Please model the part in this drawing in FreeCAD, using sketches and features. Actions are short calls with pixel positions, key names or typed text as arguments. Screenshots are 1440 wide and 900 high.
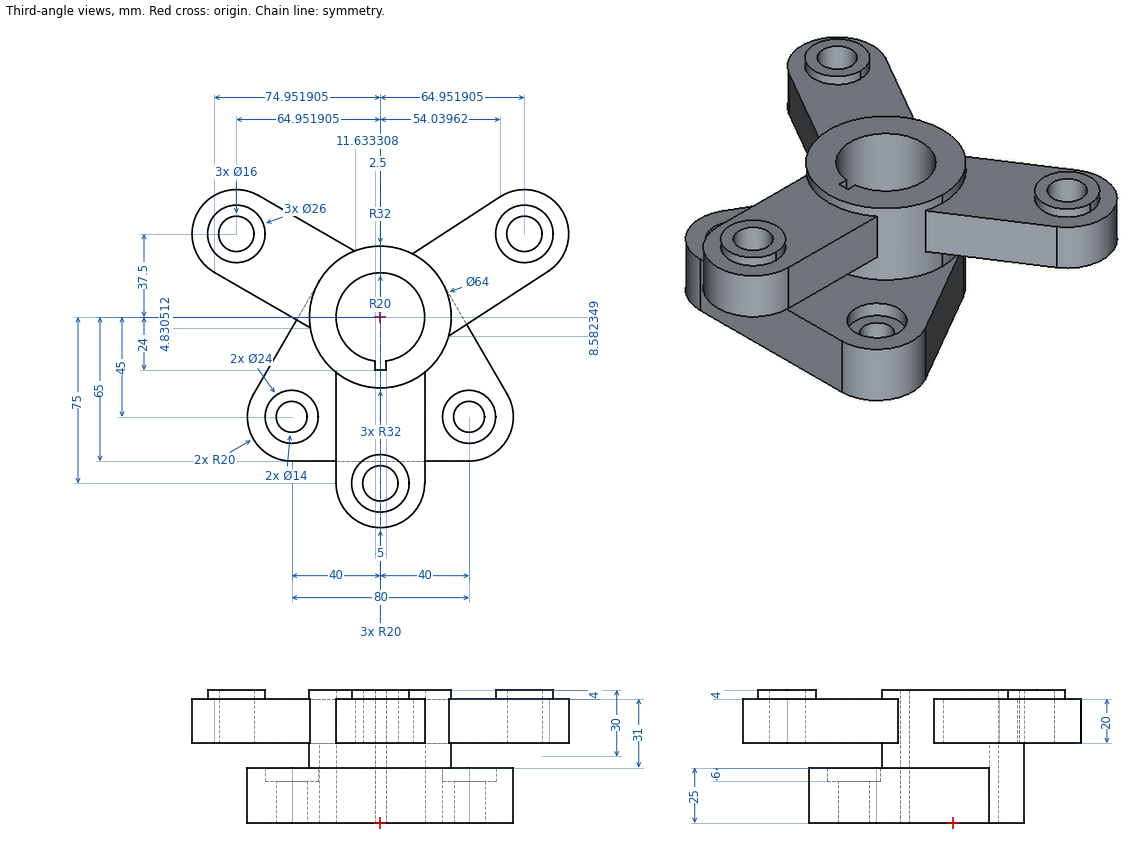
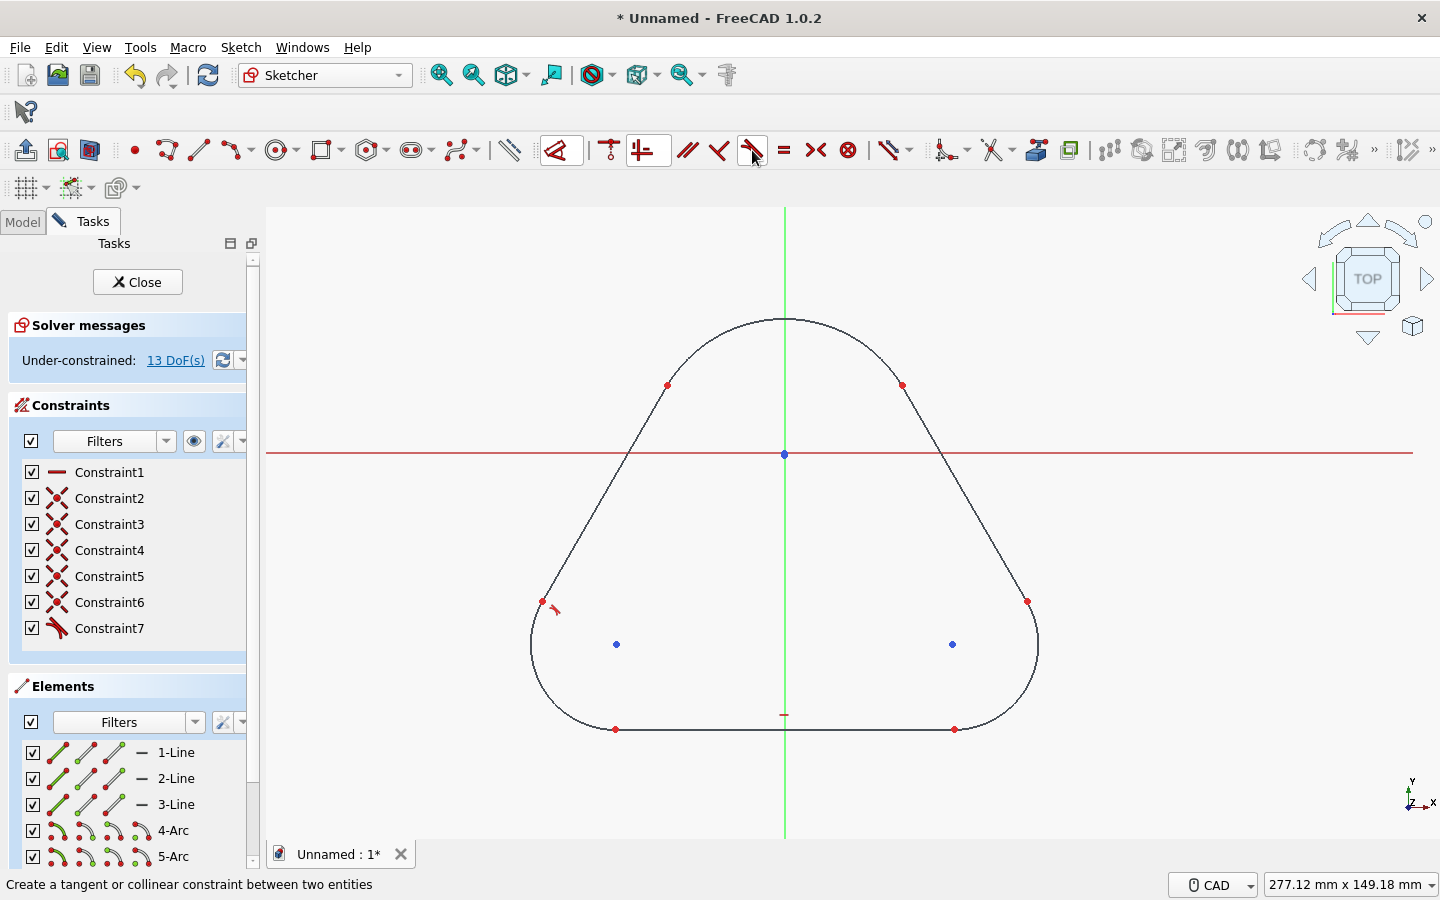
click(630, 451)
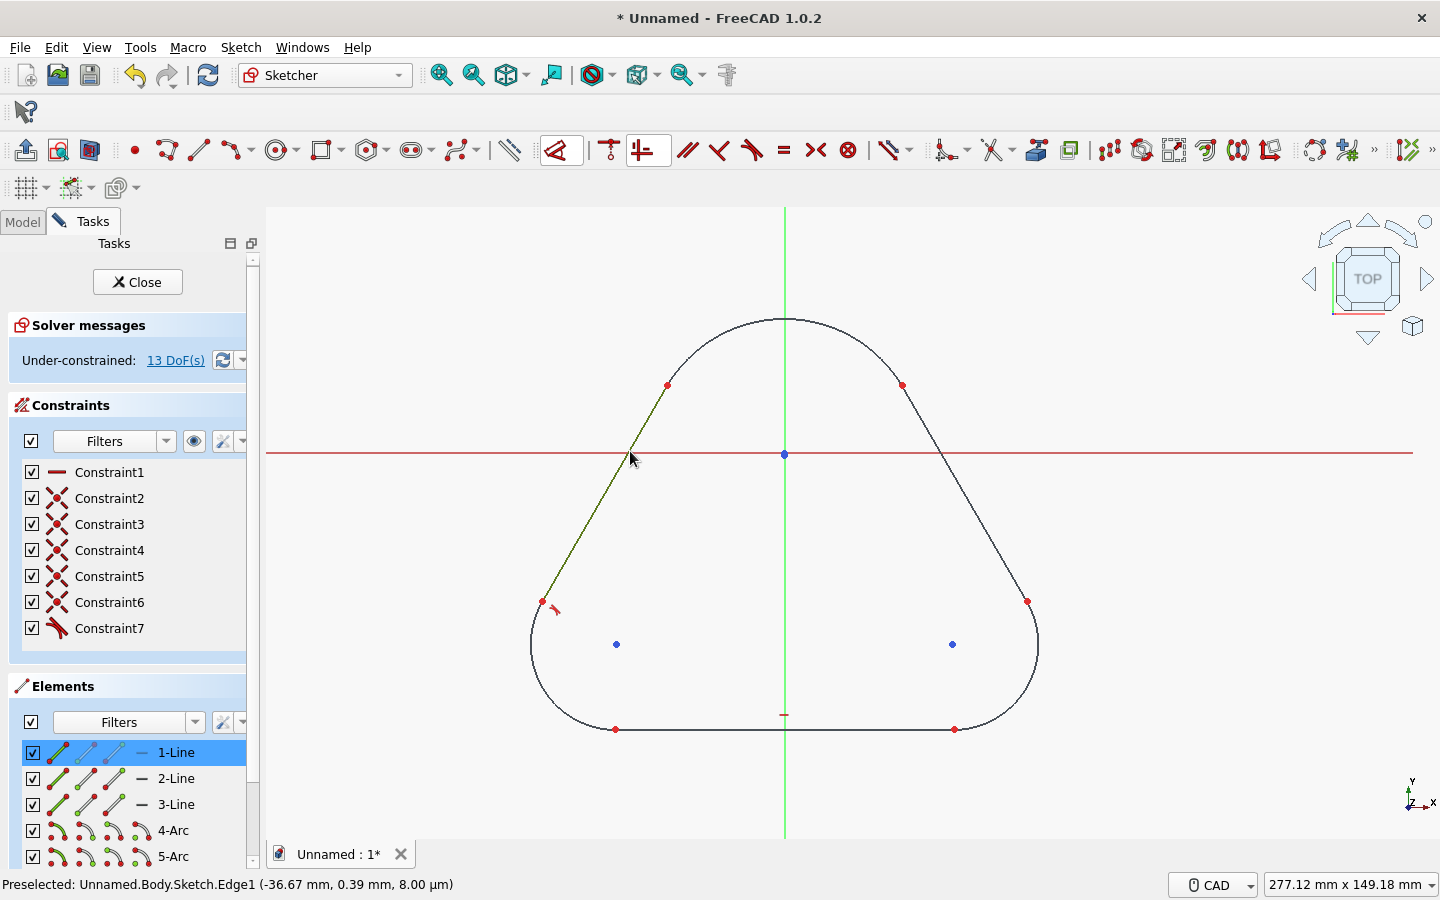
click(839, 331)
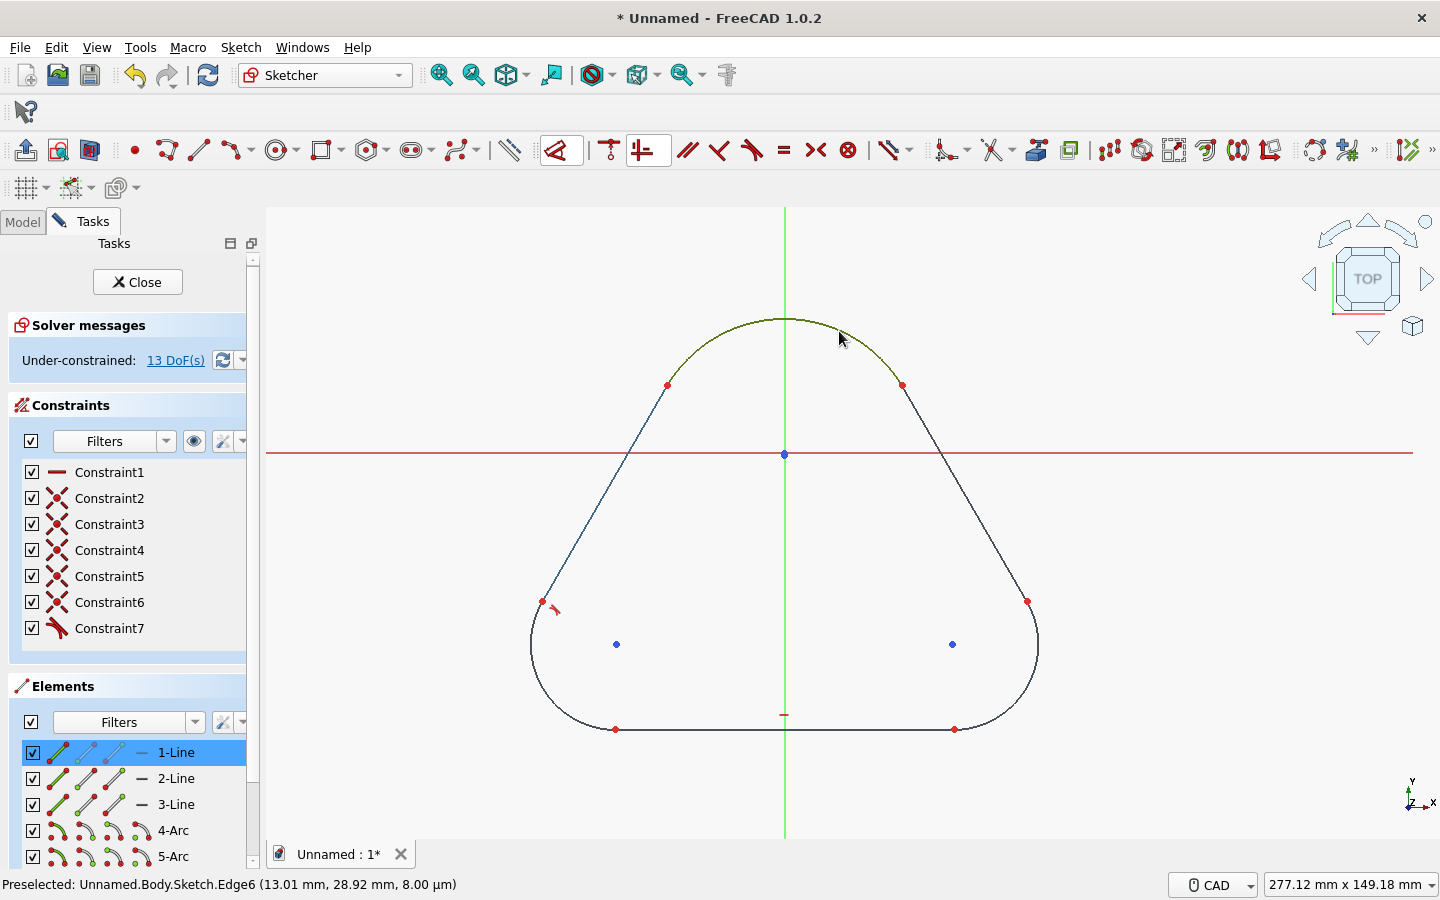
click(752, 150)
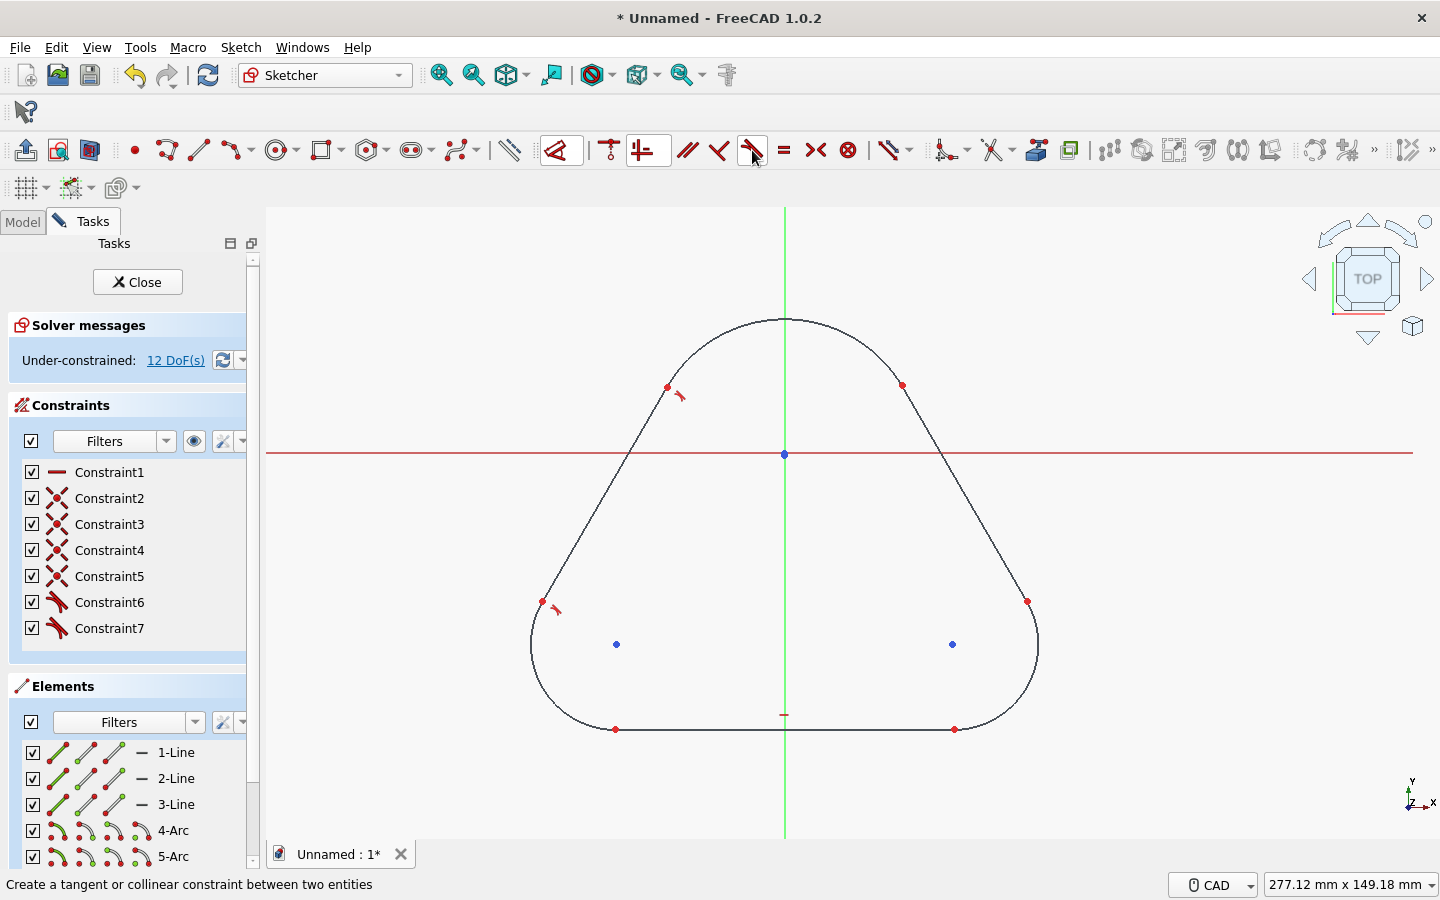
click(717, 730)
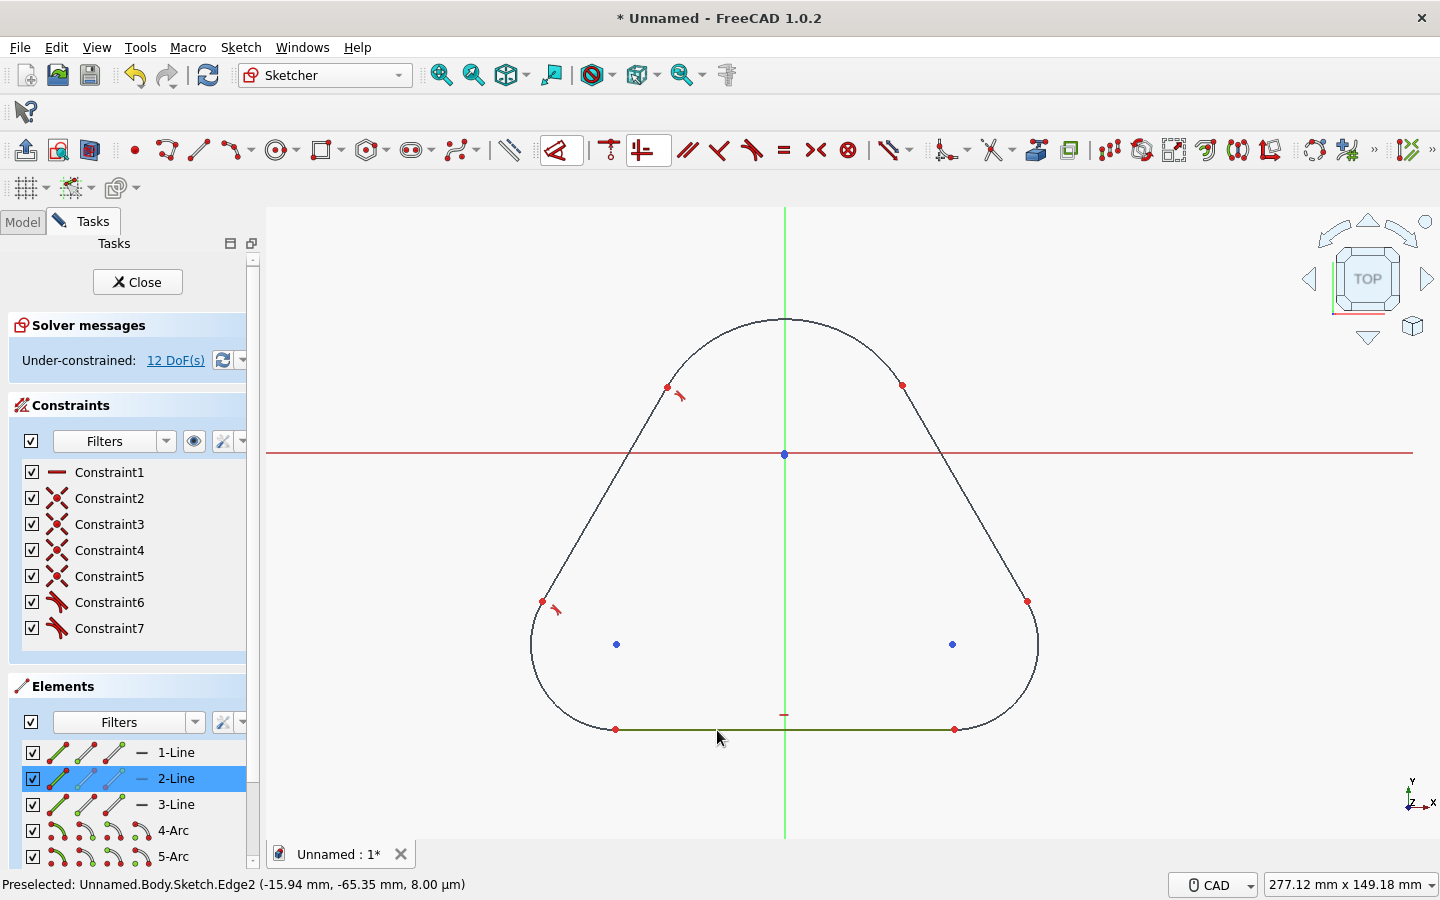
click(531, 653)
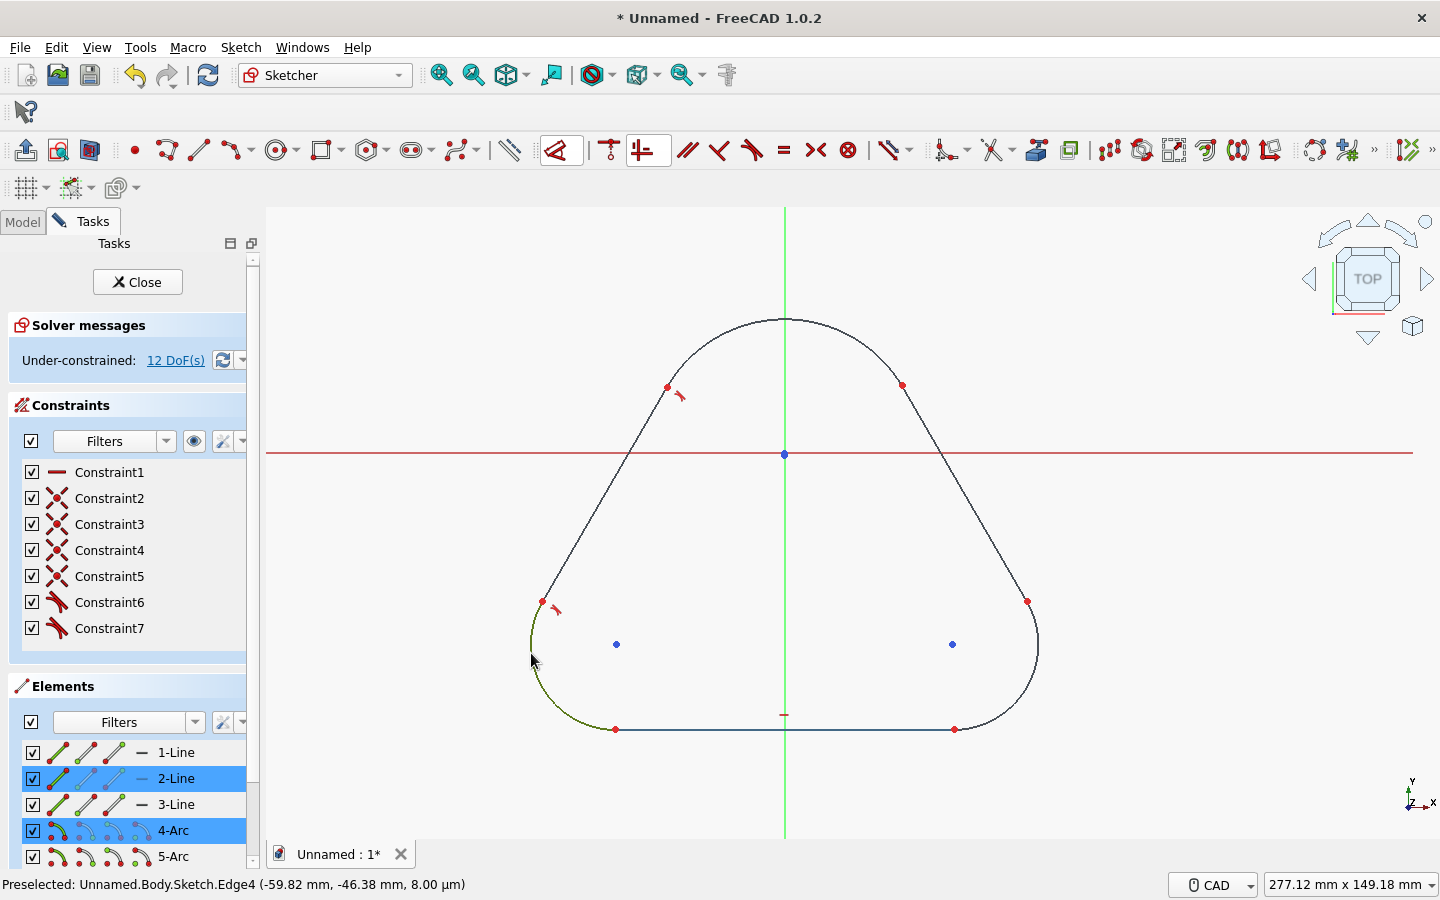
key(t)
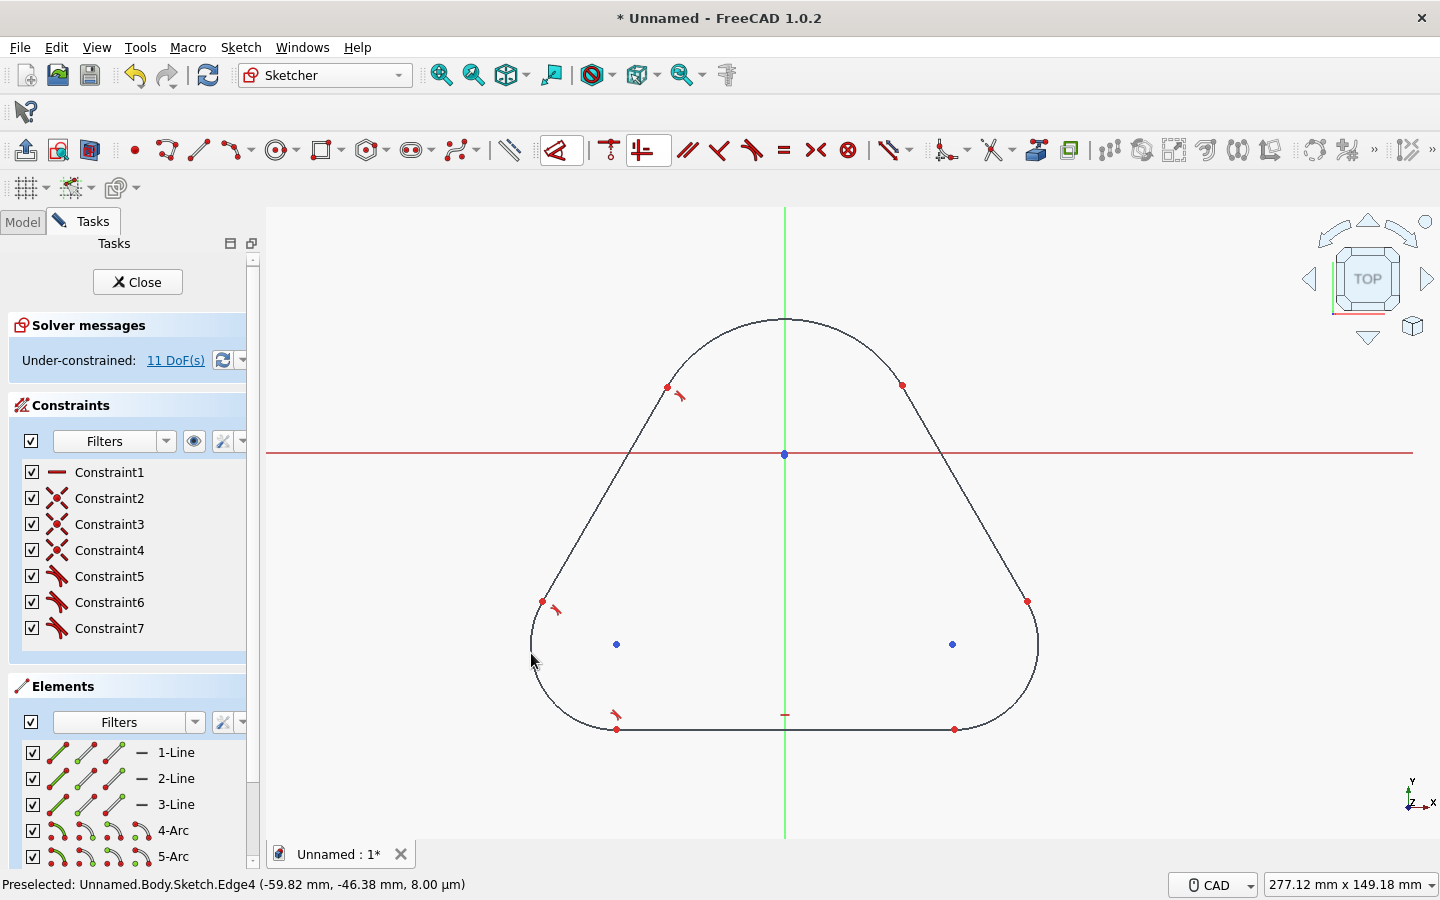
click(718, 730)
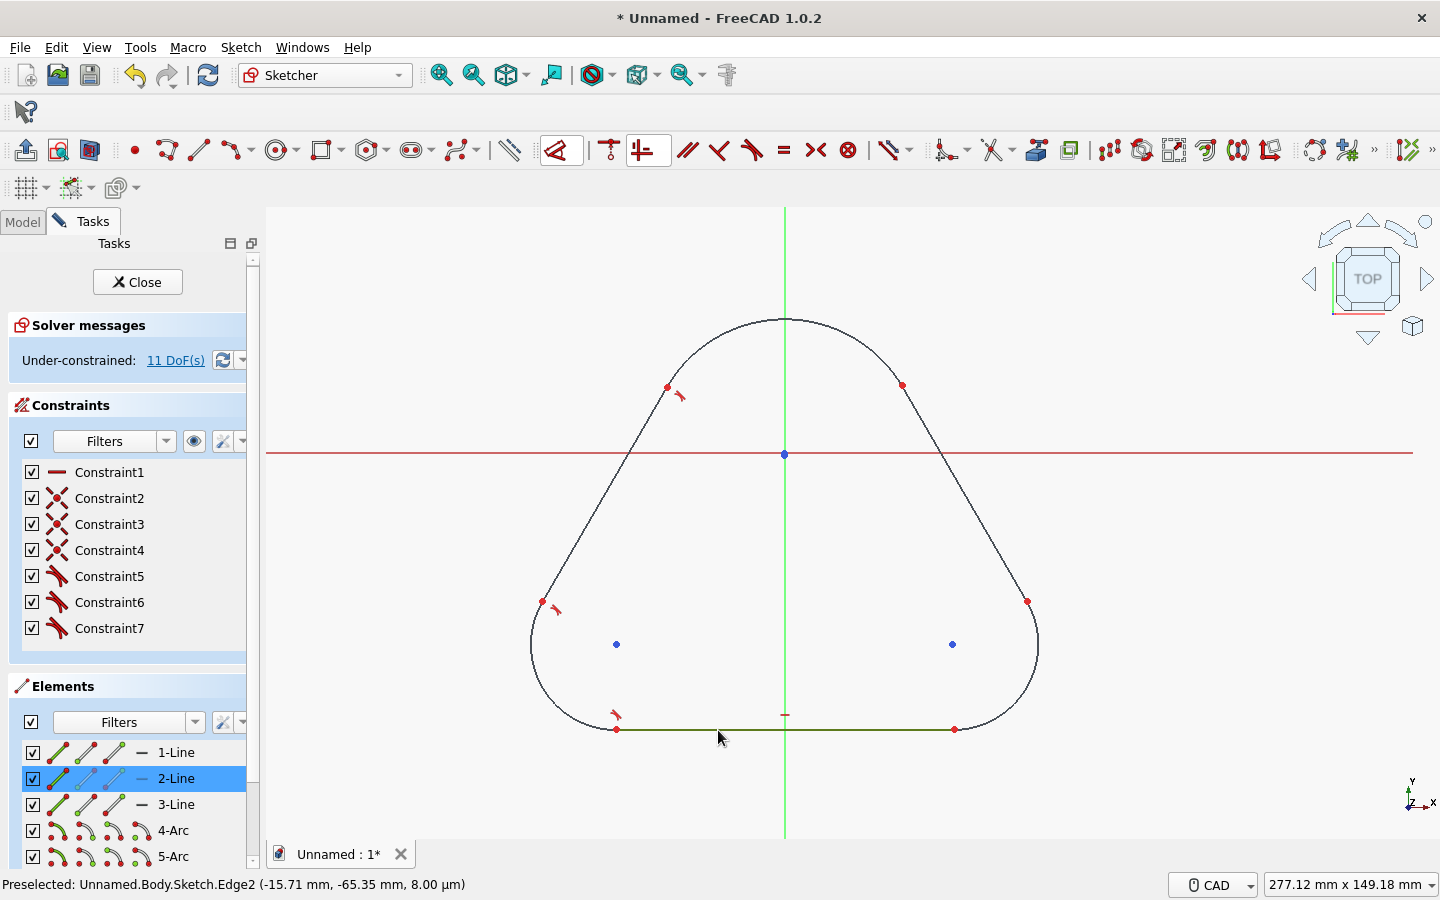
click(1004, 713)